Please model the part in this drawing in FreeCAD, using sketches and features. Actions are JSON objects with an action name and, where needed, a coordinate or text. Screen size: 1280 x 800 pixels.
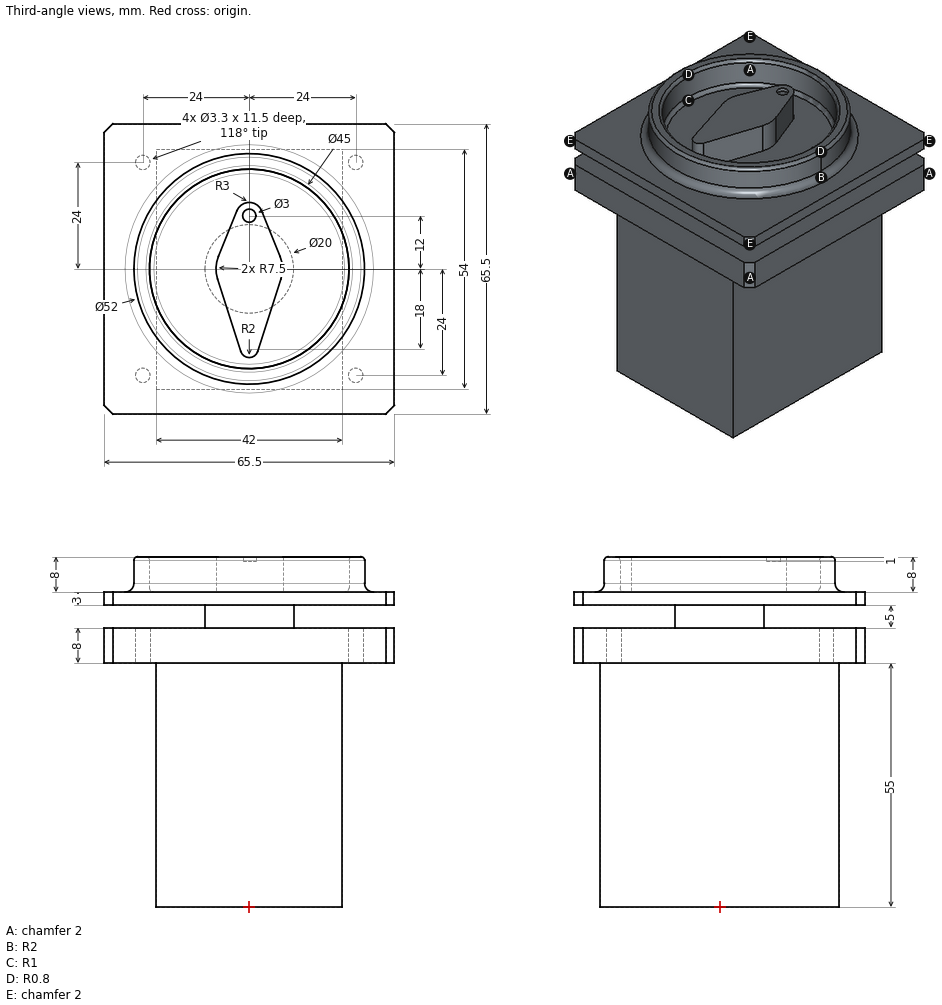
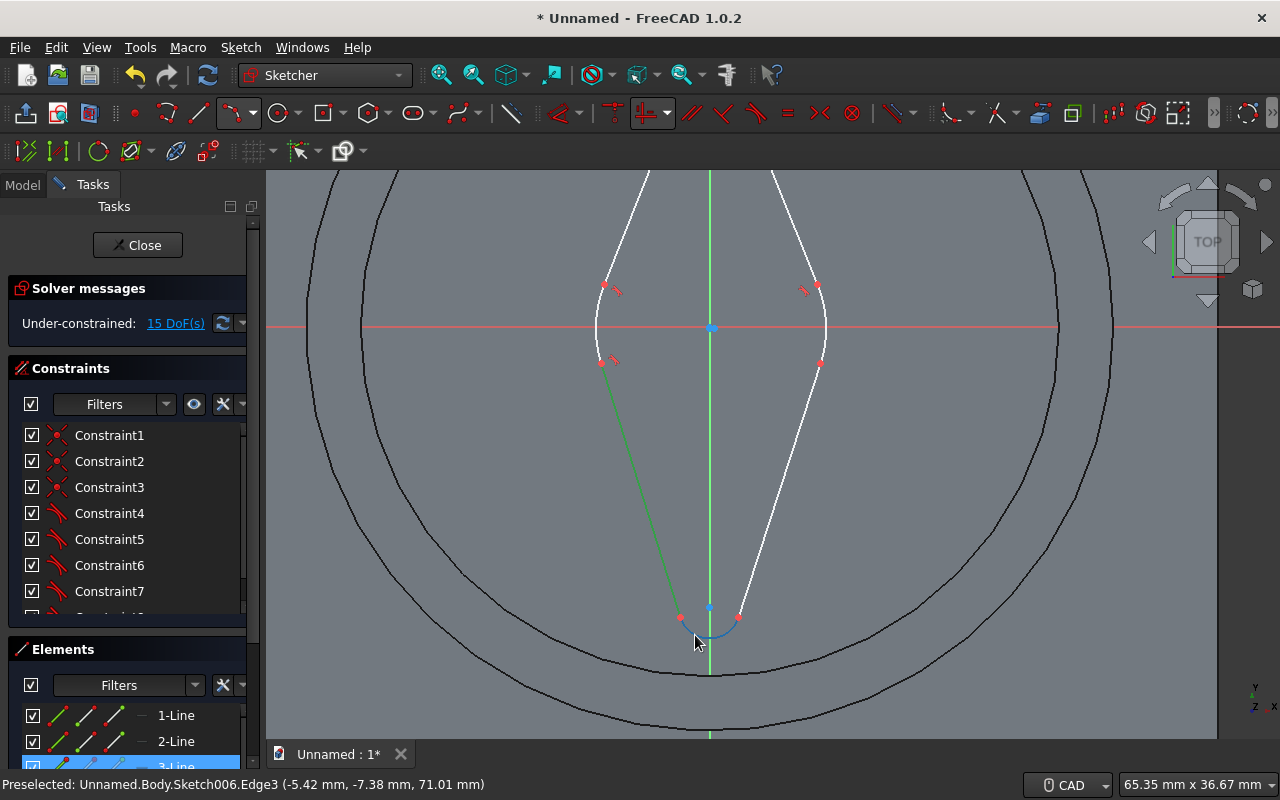
{"action": "left_click", "coordinate": [695, 635]}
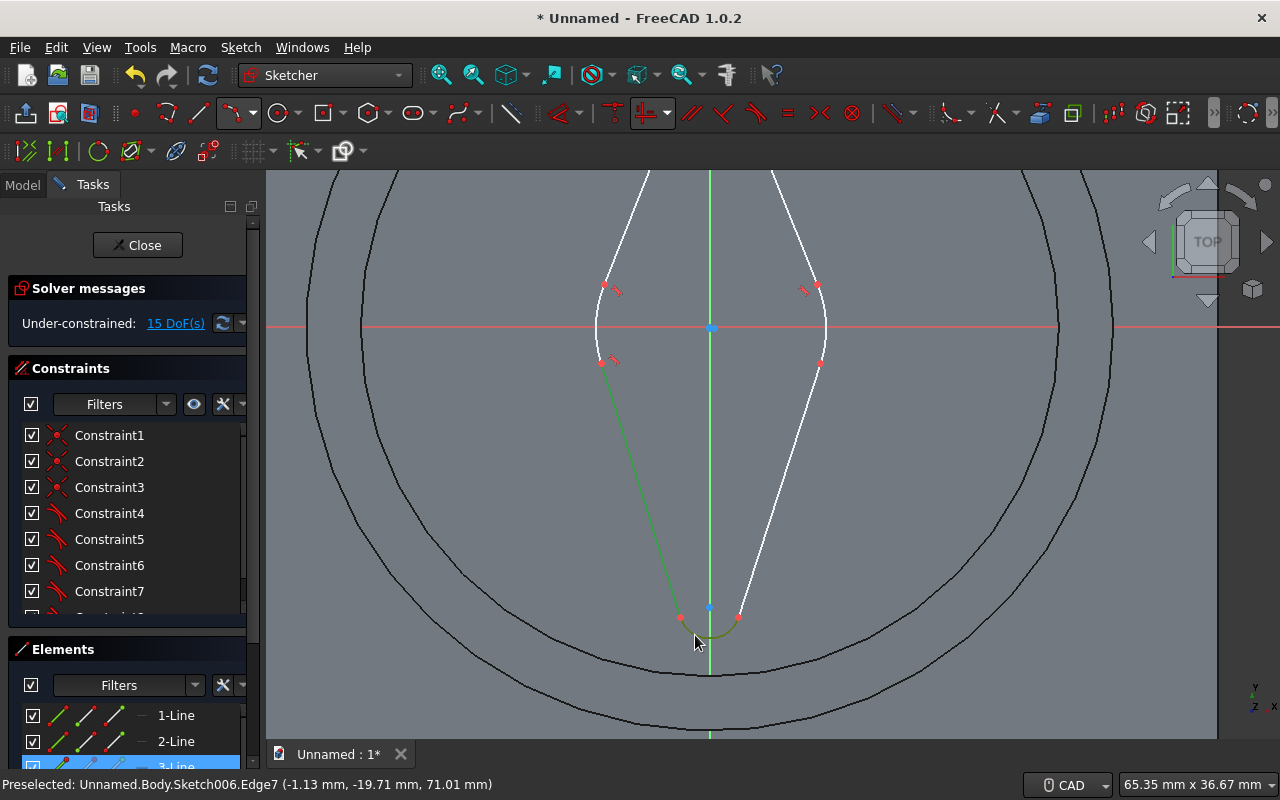
{"action": "left_click", "coordinate": [756, 114]}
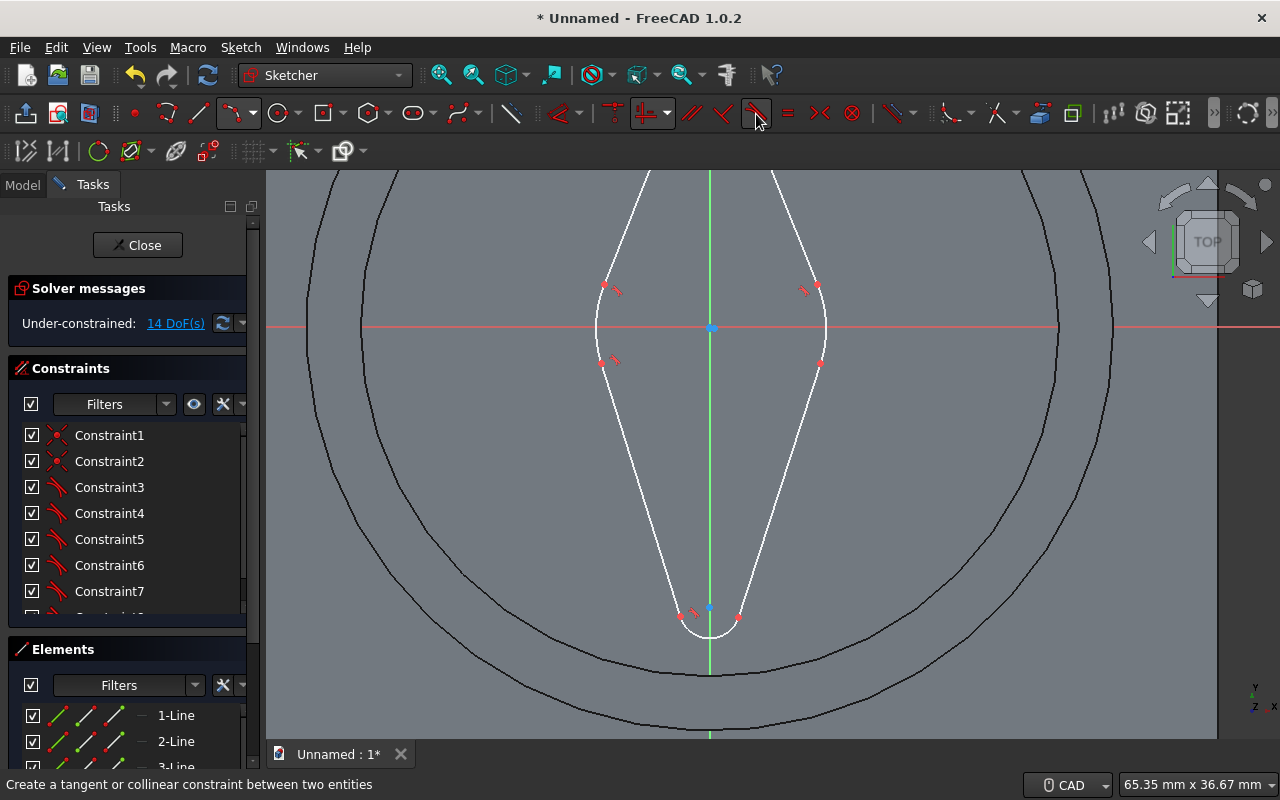
{"action": "left_click", "coordinate": [763, 541]}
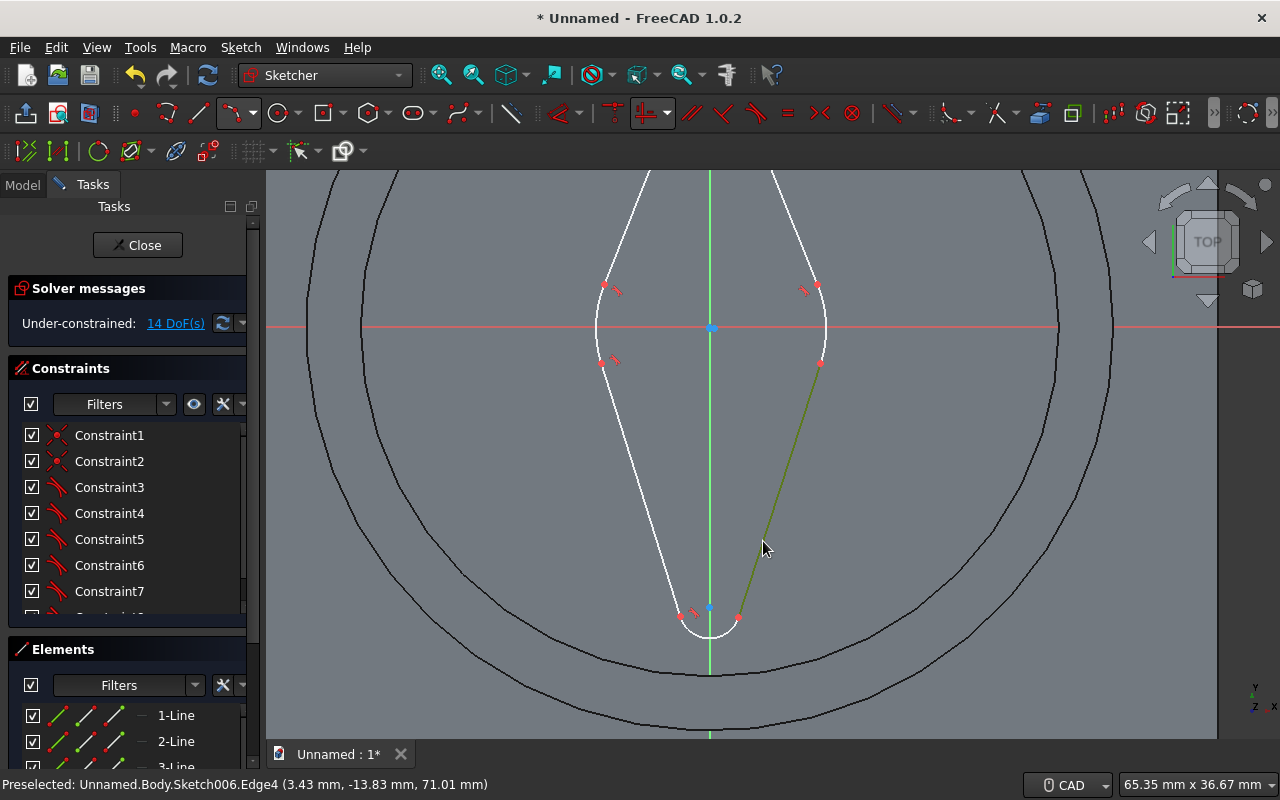
{"action": "left_click", "coordinate": [695, 634]}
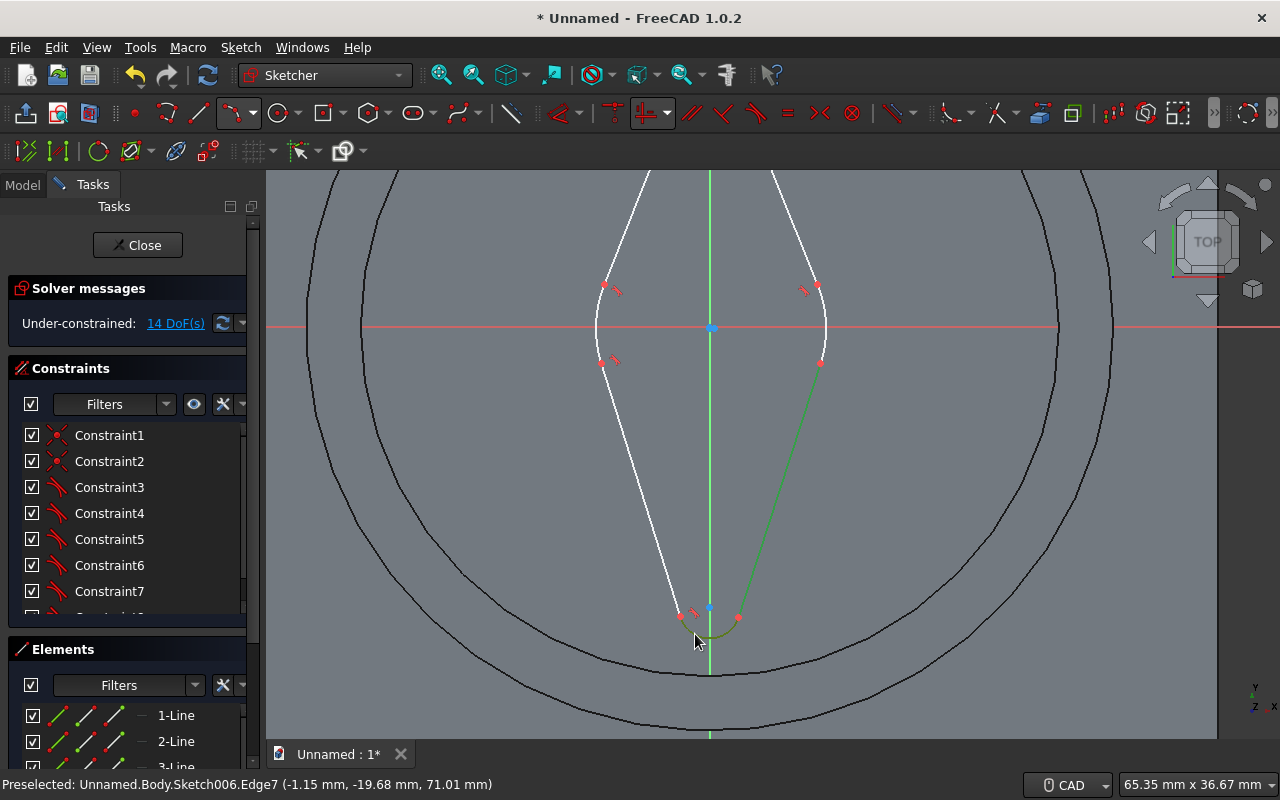
{"action": "left_click", "coordinate": [756, 114]}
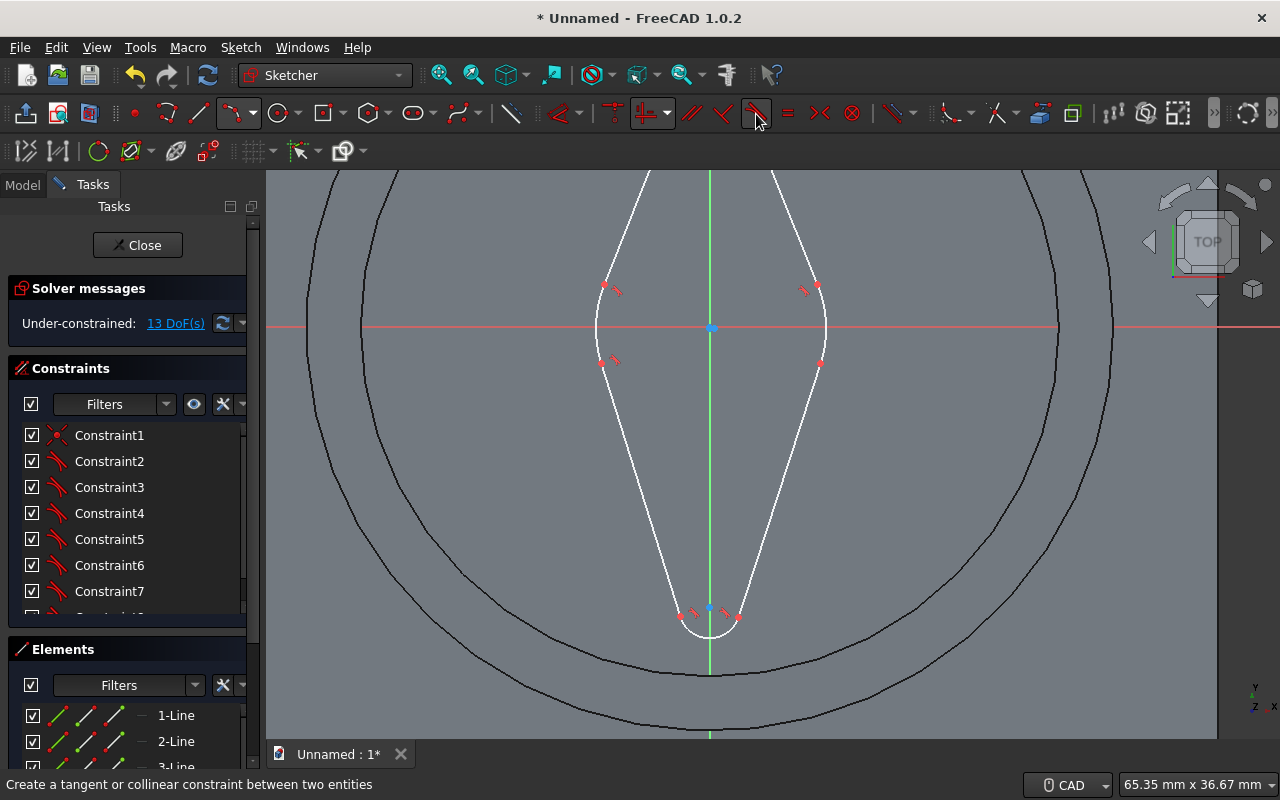
{"action": "left_click", "coordinate": [763, 541]}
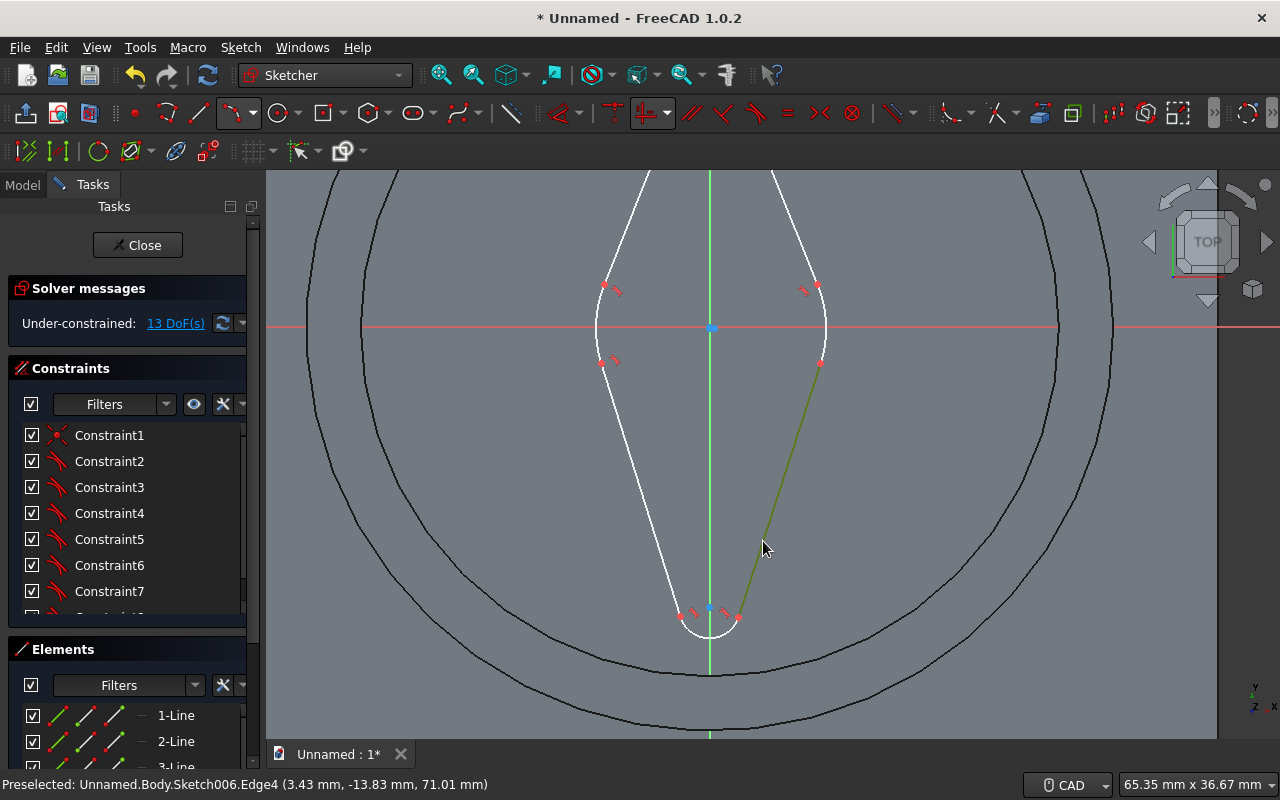
{"action": "left_click", "coordinate": [826, 340]}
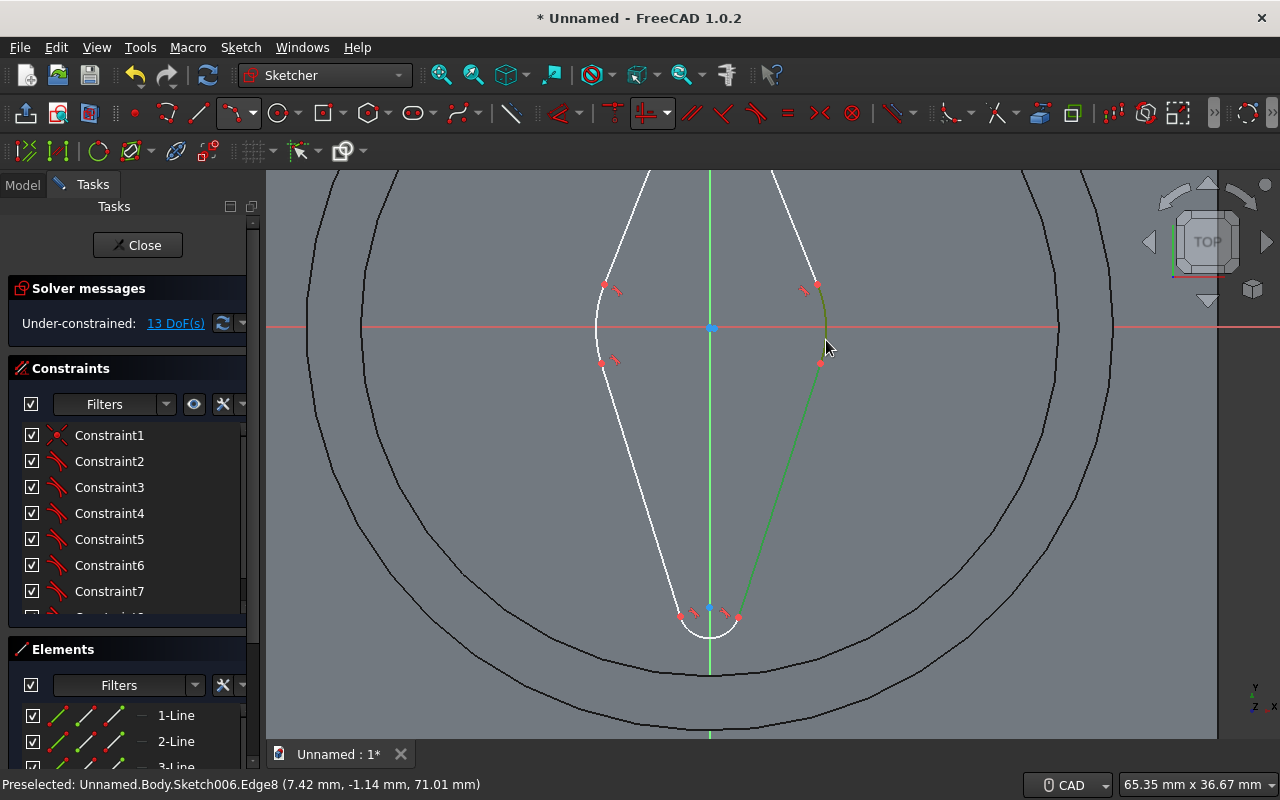
{"action": "left_click", "coordinate": [756, 114]}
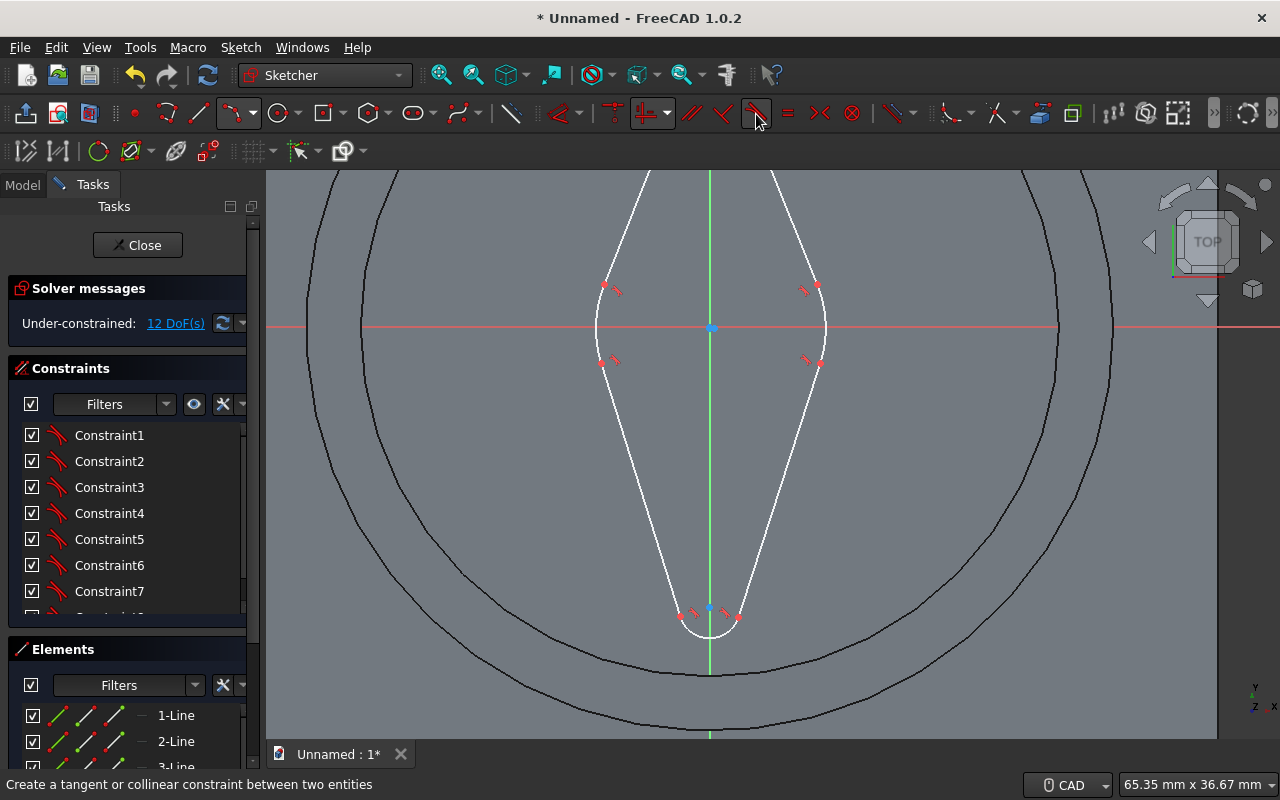
{"action": "left_click", "coordinate": [598, 308]}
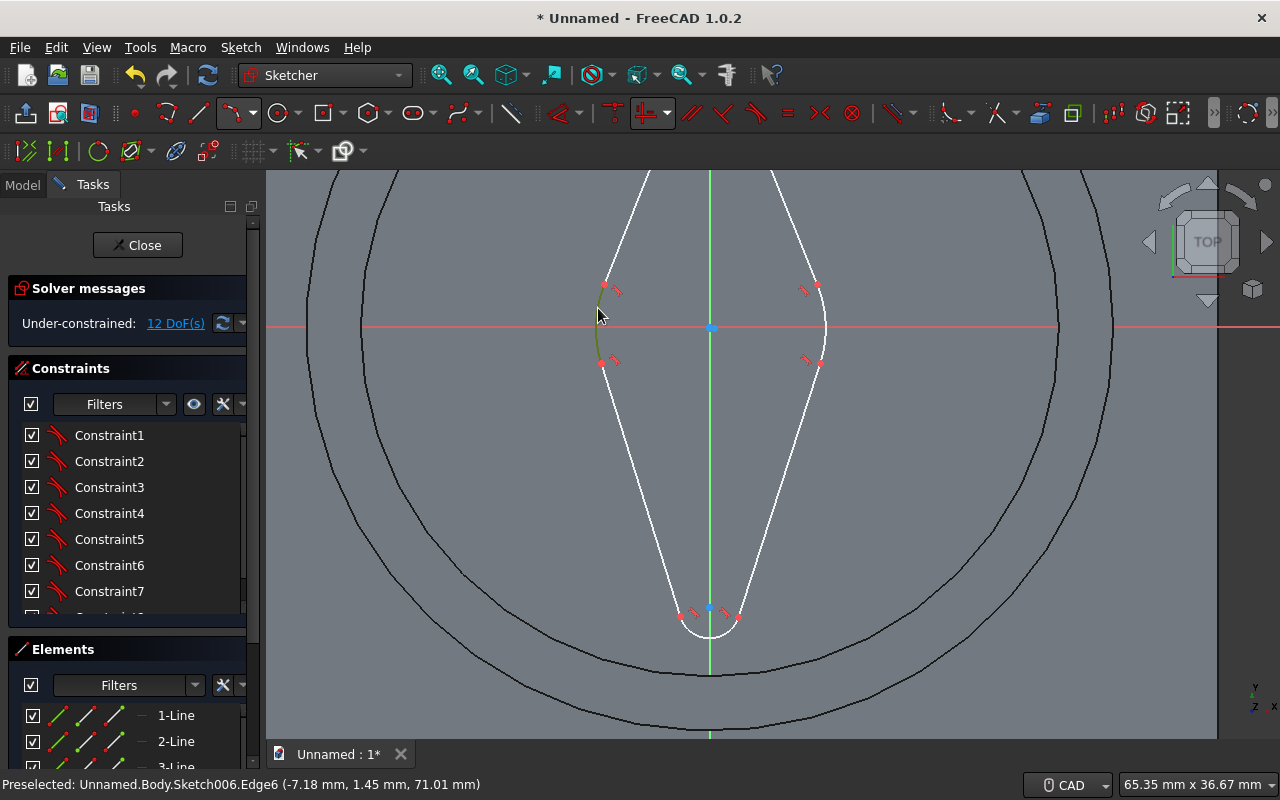
{"action": "left_click", "coordinate": [825, 340]}